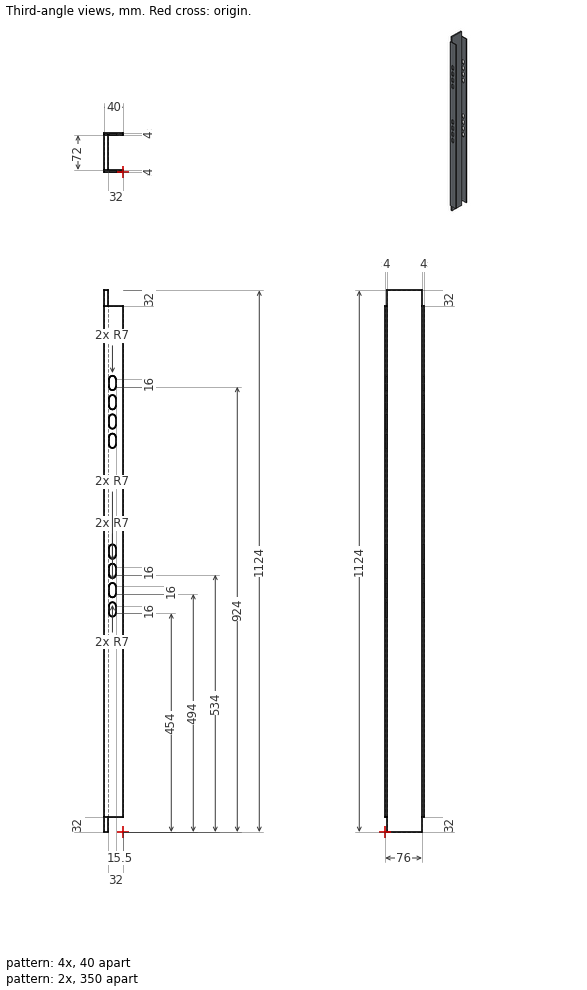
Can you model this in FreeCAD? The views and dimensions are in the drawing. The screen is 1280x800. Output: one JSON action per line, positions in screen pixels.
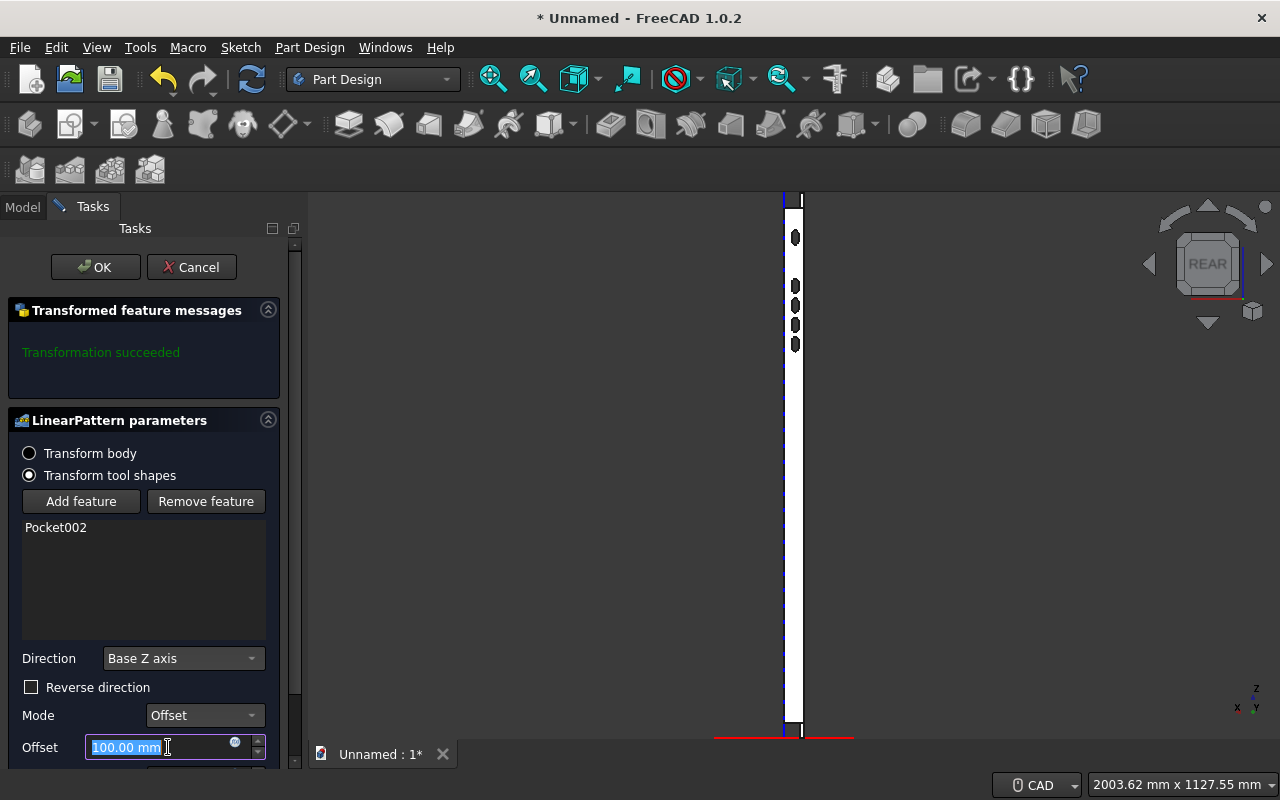
{"action": "type", "text": "350"}
{"action": "key", "text": "Tab"}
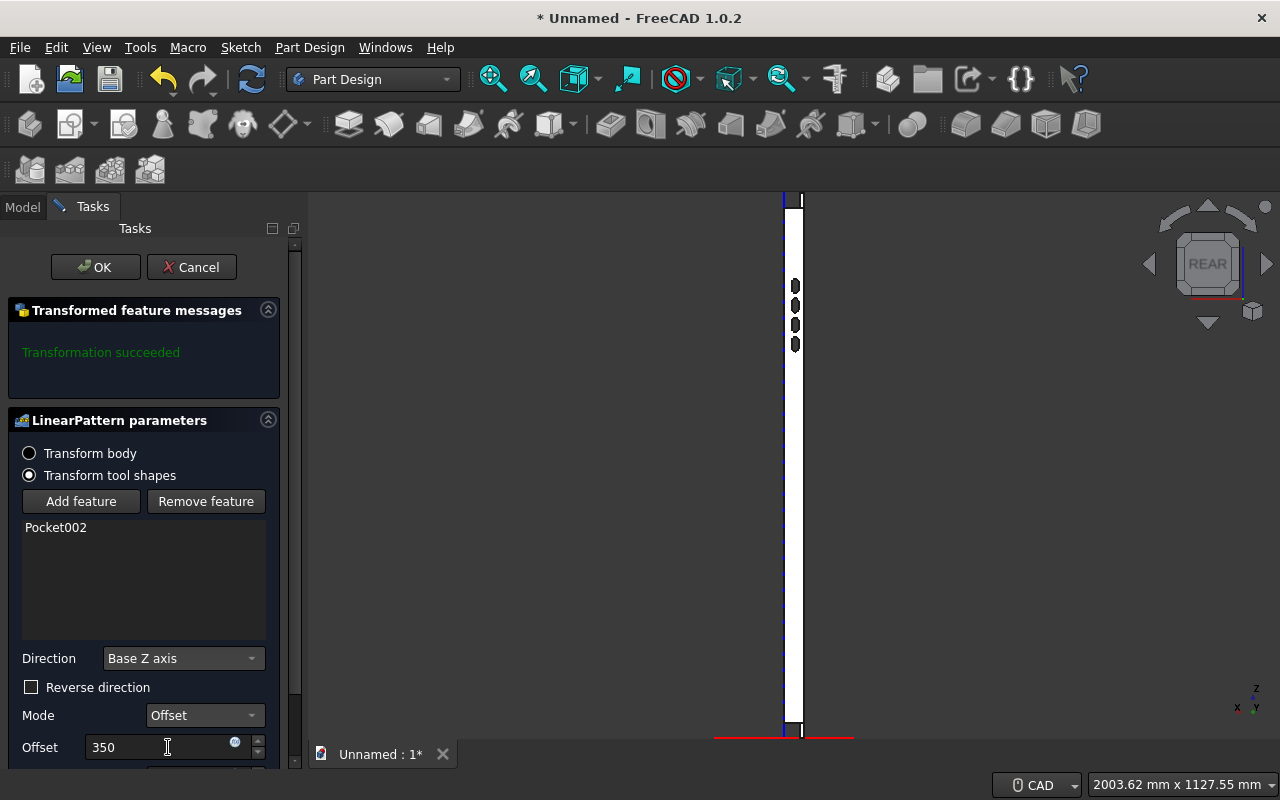
{"action": "scroll", "coordinate": [295, 503], "scroll_direction": "down", "scroll_amount": 2}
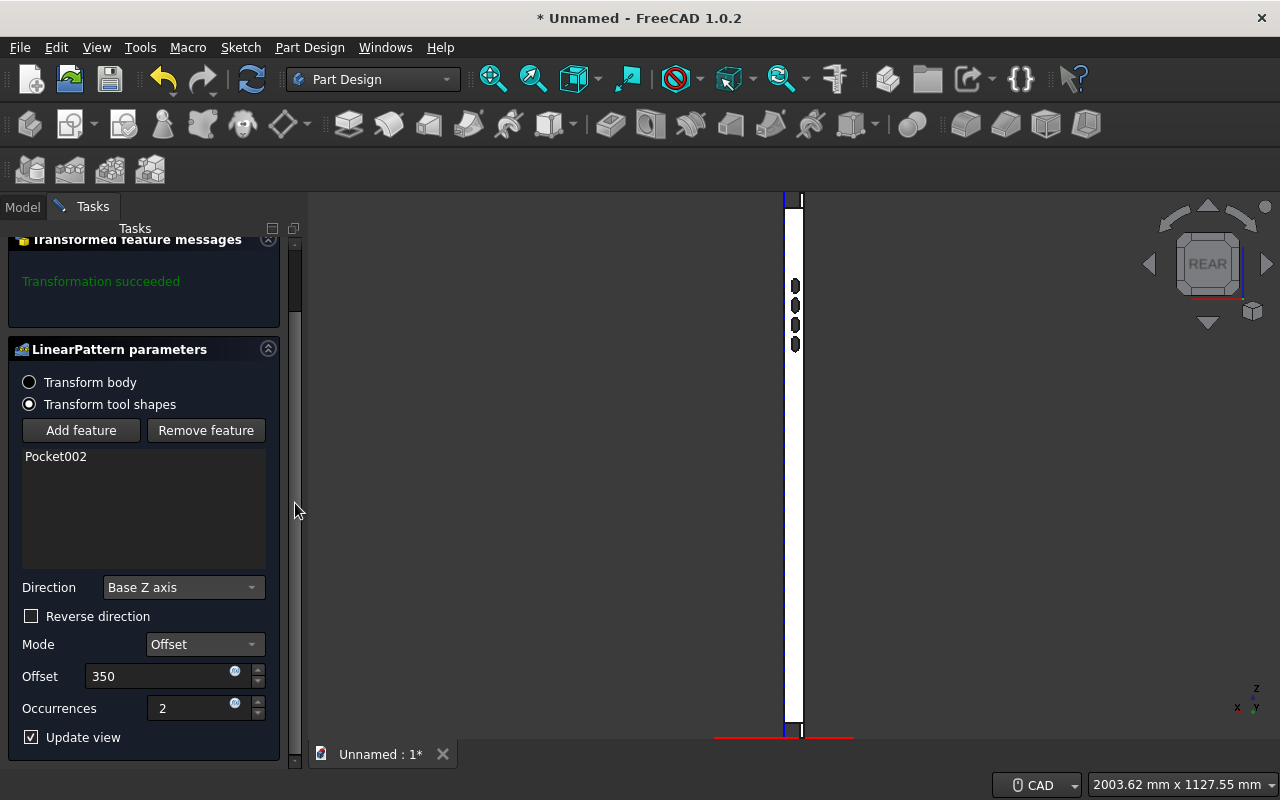
{"action": "triple_click", "coordinate": [198, 708]}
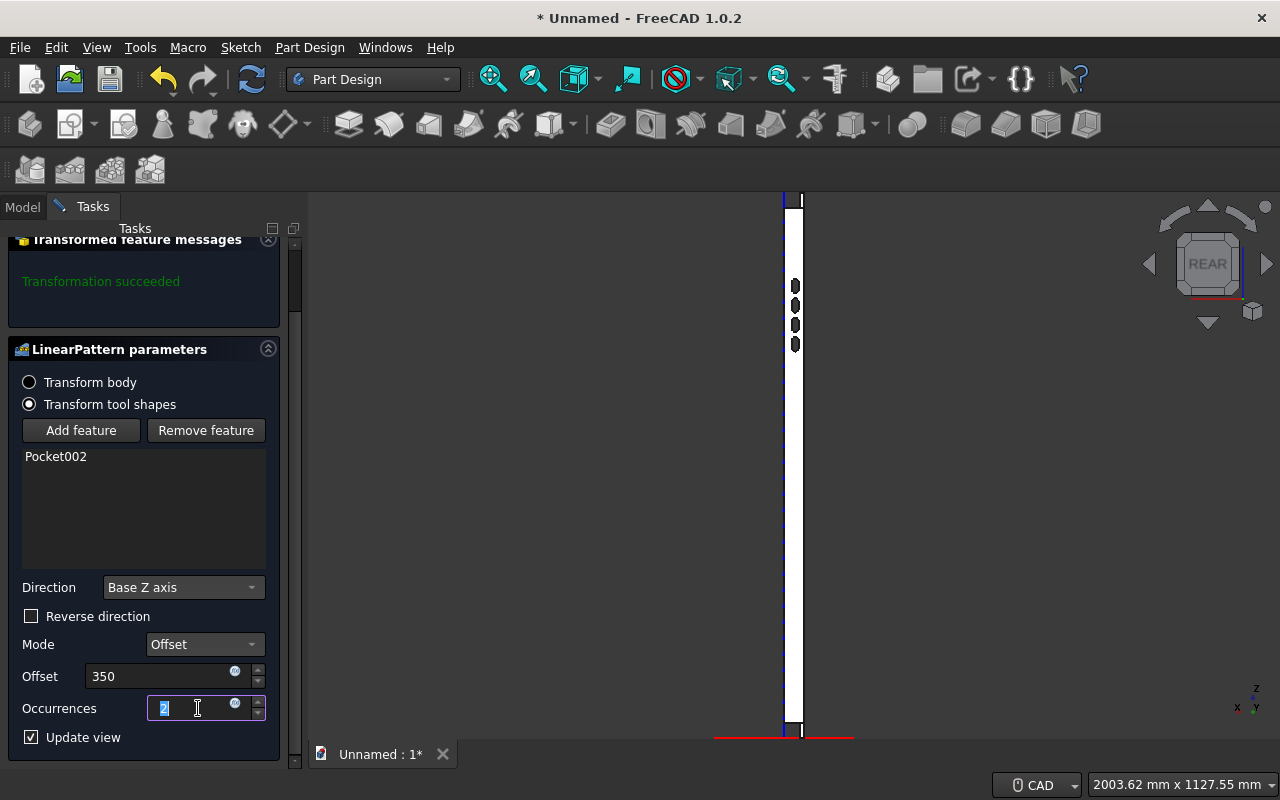
{"action": "type", "text": "2"}
{"action": "key", "text": "Tab"}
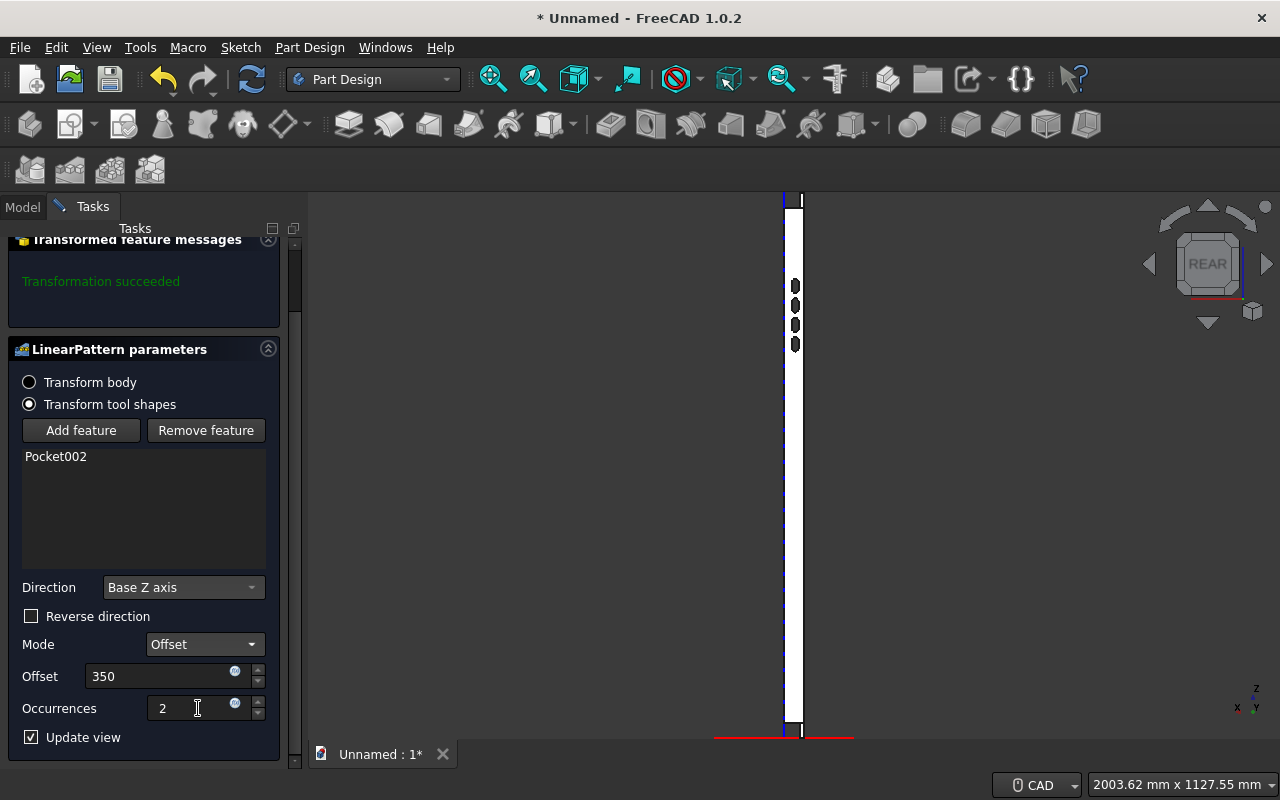
{"action": "left_click", "coordinate": [30, 616]}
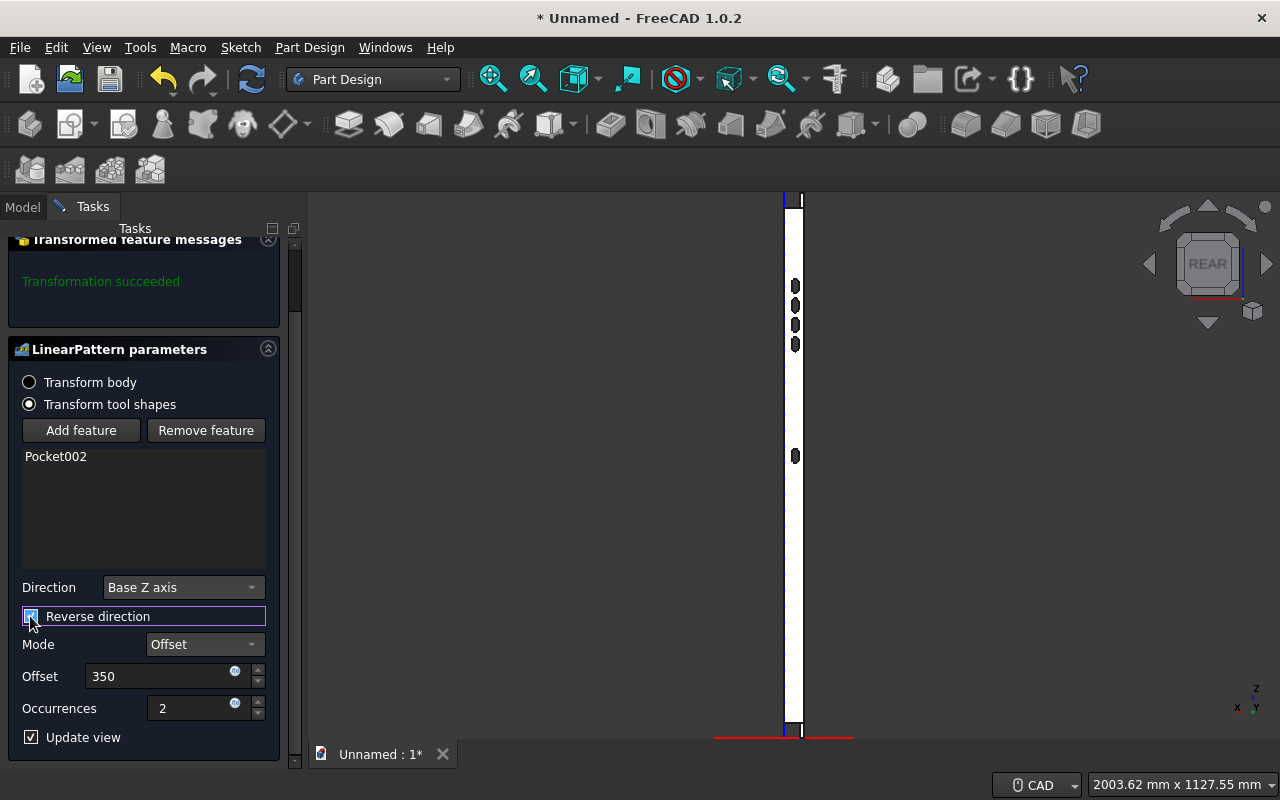
{"action": "scroll", "coordinate": [295, 503], "scroll_direction": "up", "scroll_amount": 2}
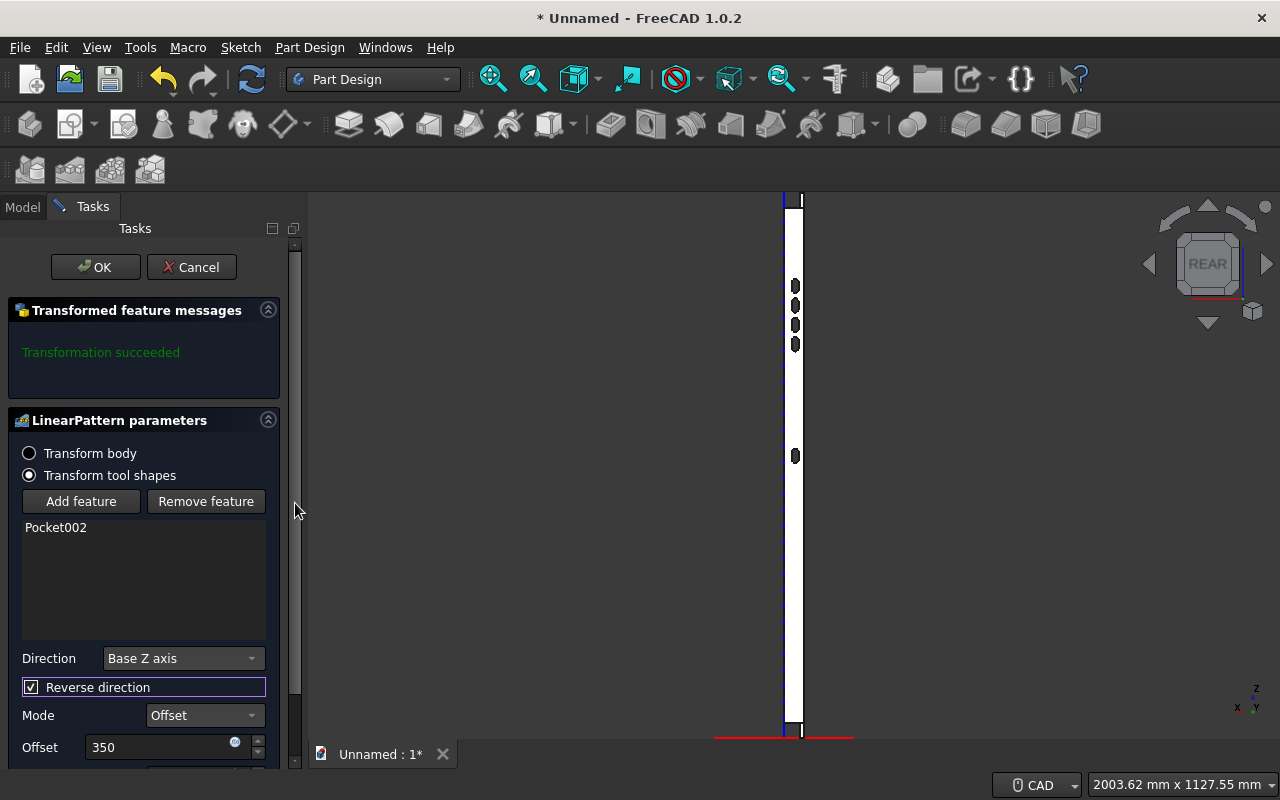
{"action": "left_click", "coordinate": [96, 267]}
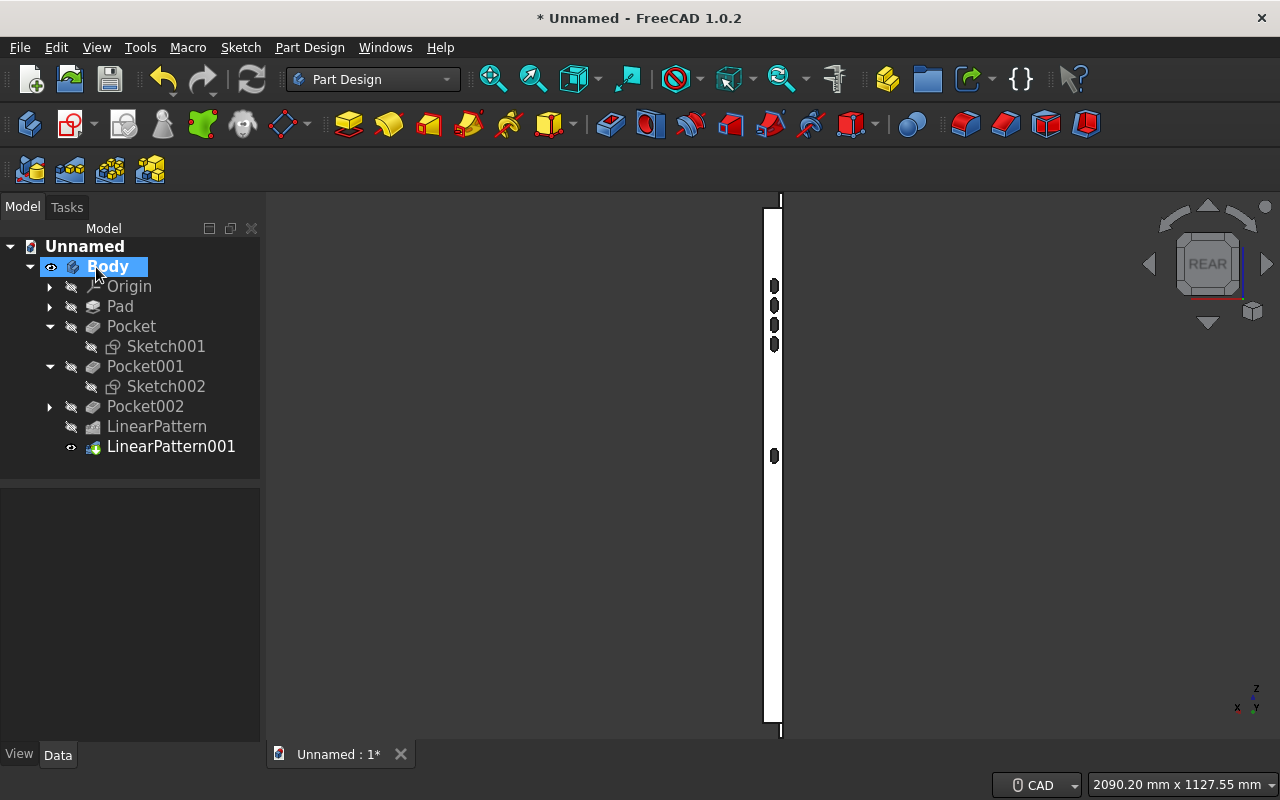
{"action": "left_click", "coordinate": [773, 244]}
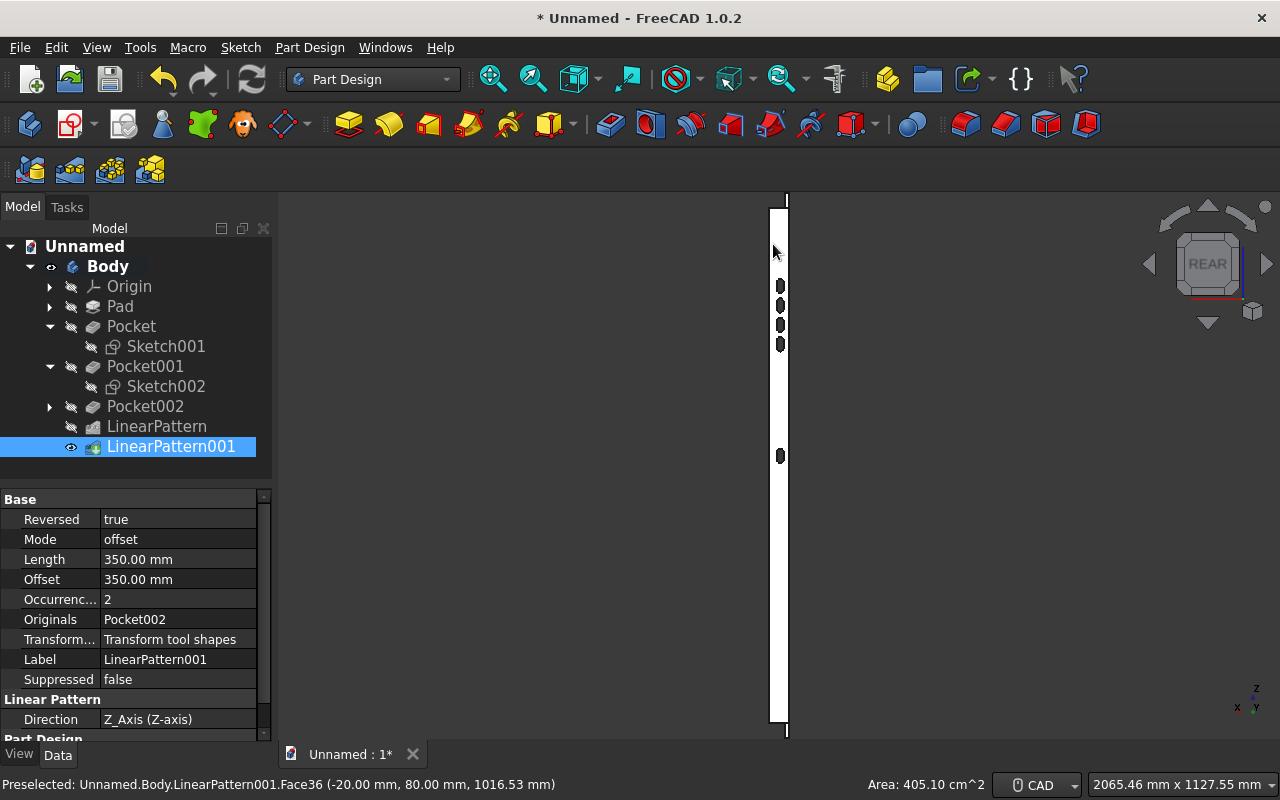
{"action": "left_click", "coordinate": [70, 124]}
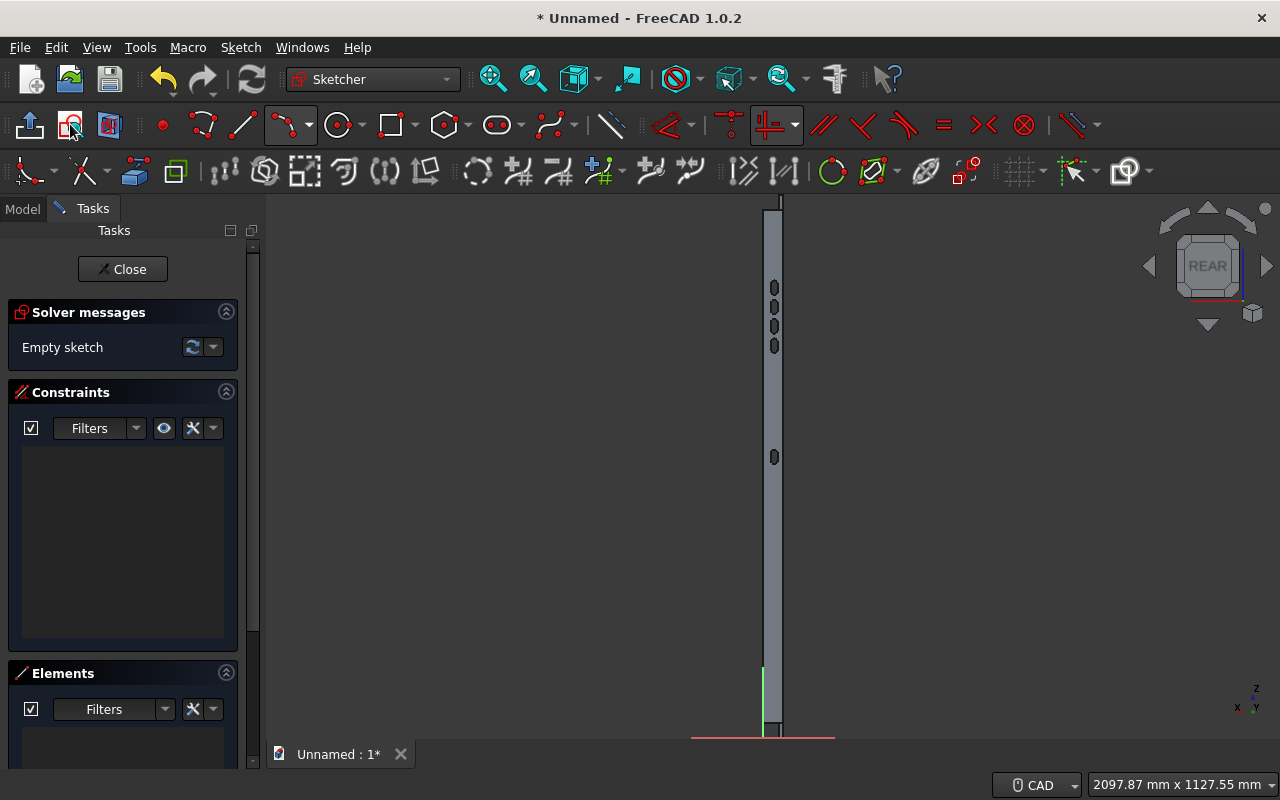
{"action": "scroll", "coordinate": [778, 477], "scroll_direction": "up", "scroll_amount": 15}